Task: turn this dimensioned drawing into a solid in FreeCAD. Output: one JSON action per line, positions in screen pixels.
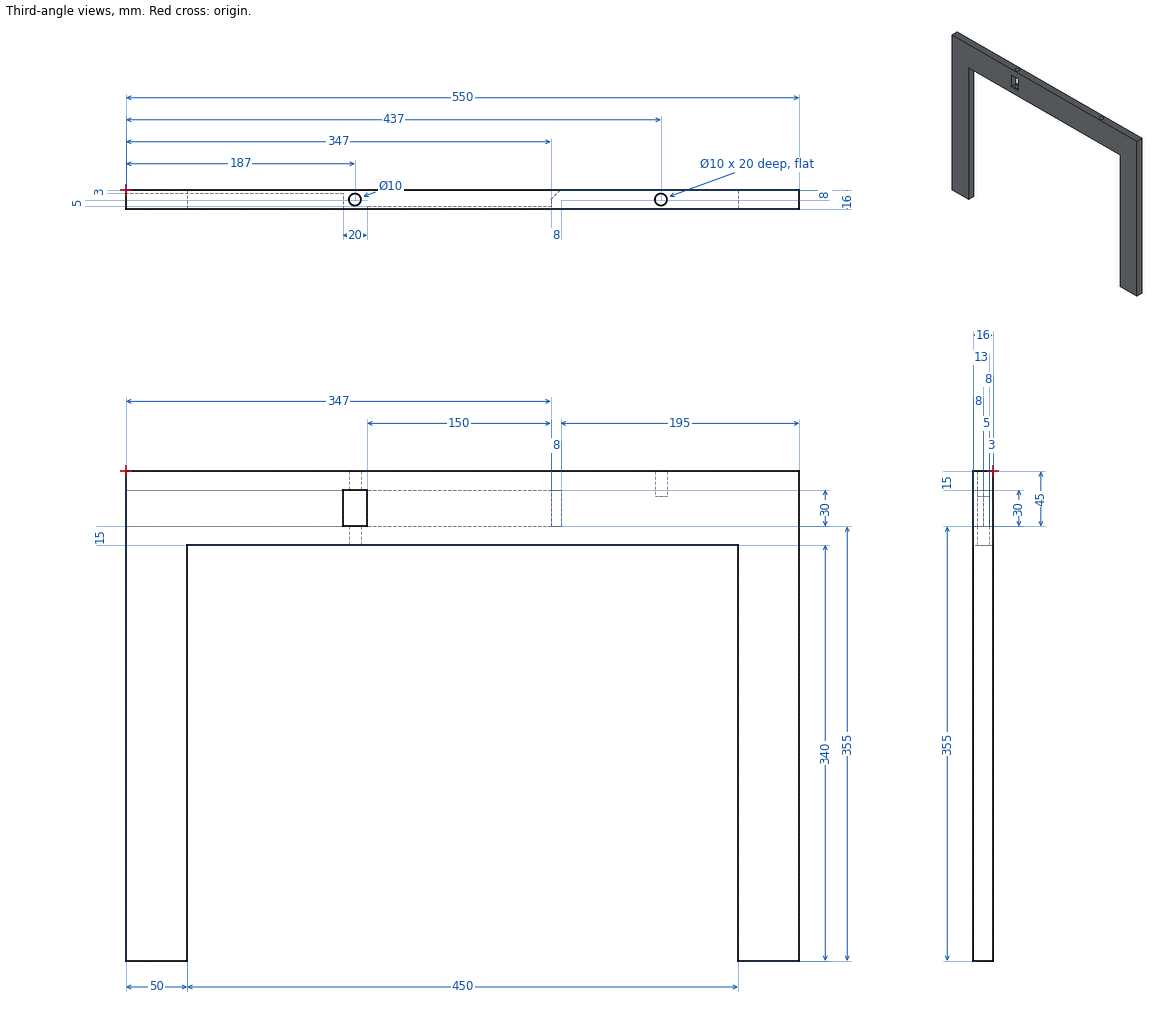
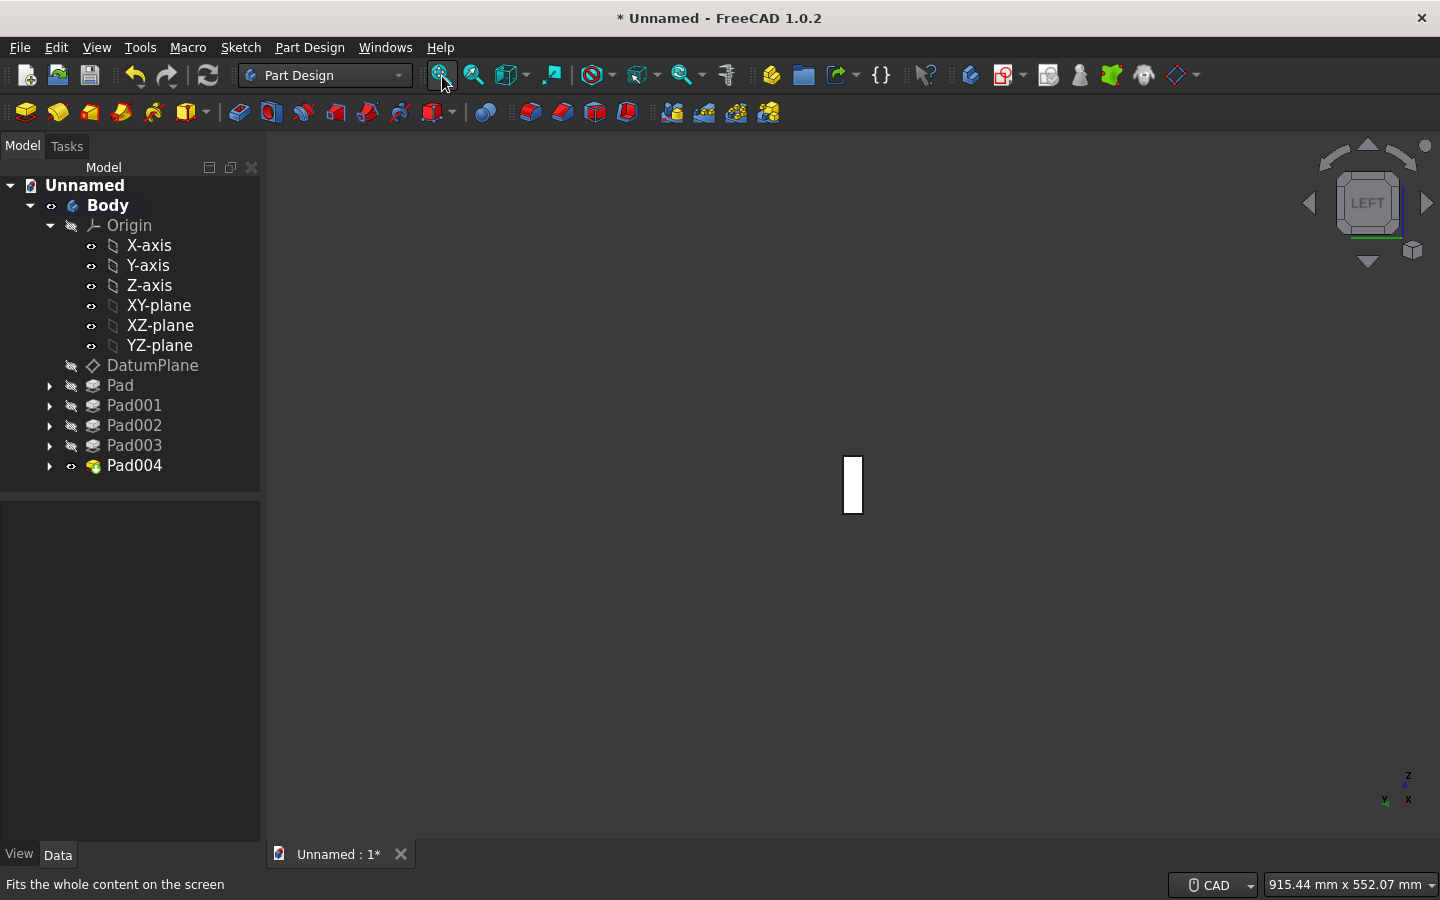
{"action": "key", "text": "4"}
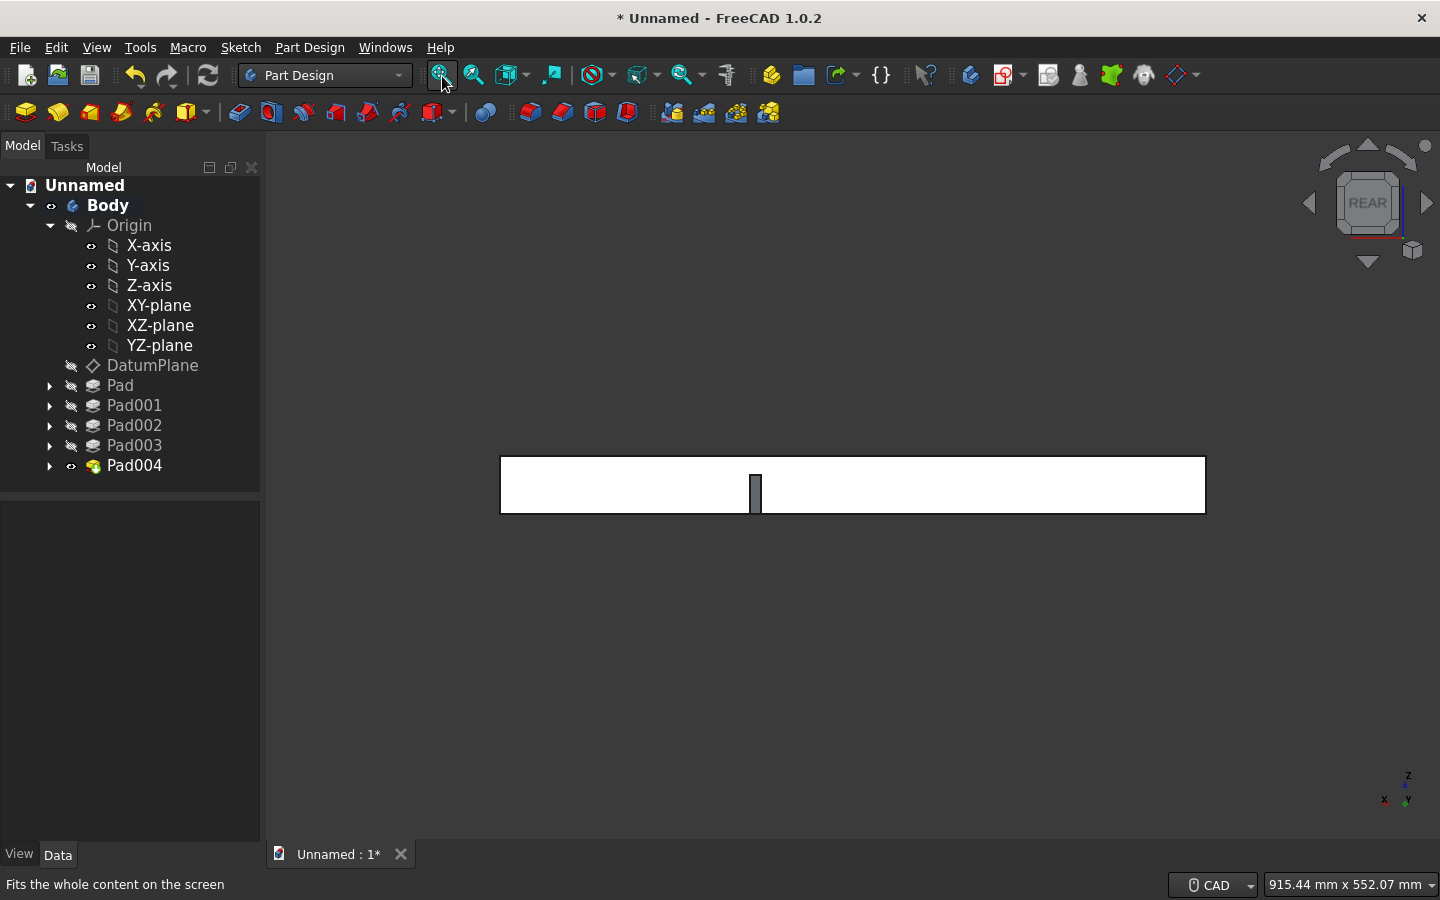
{"action": "left_click", "coordinate": [551, 484]}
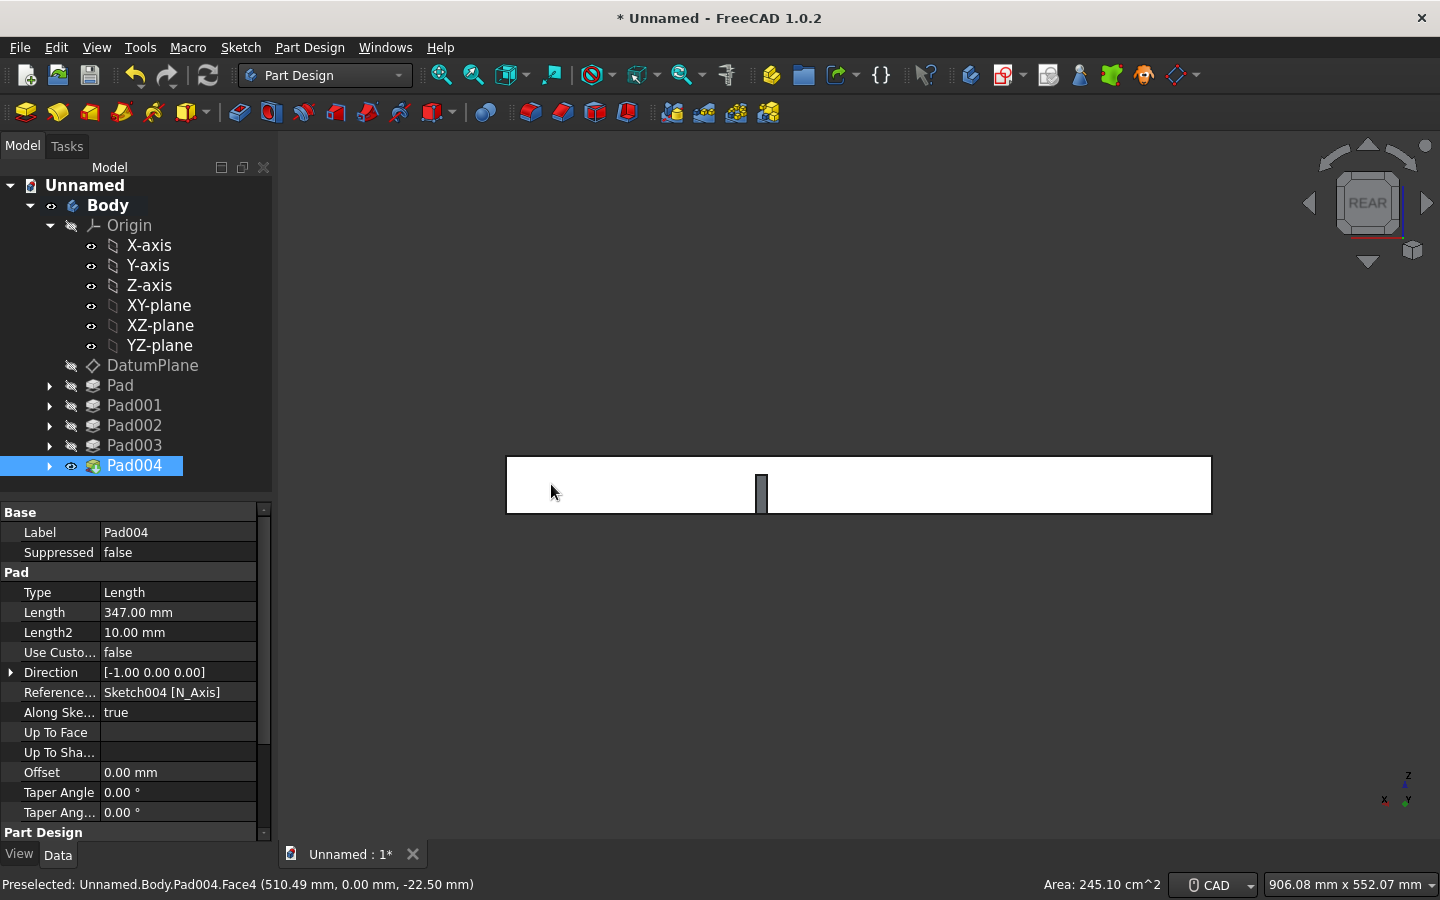
{"action": "left_click", "coordinate": [1004, 76]}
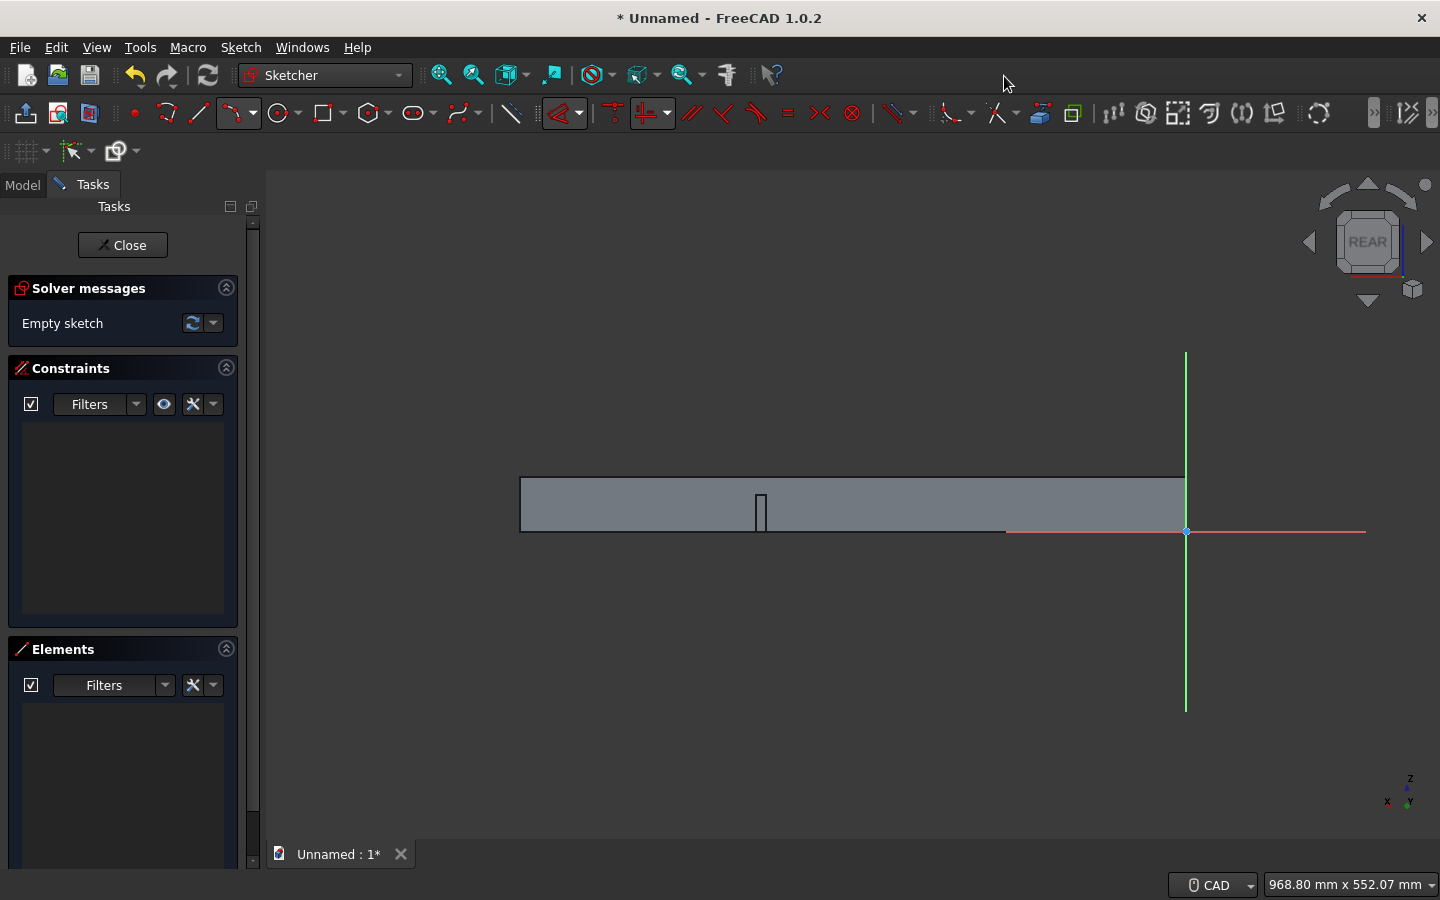
{"action": "scroll", "coordinate": [1275, 532], "scroll_direction": "up", "scroll_amount": 2}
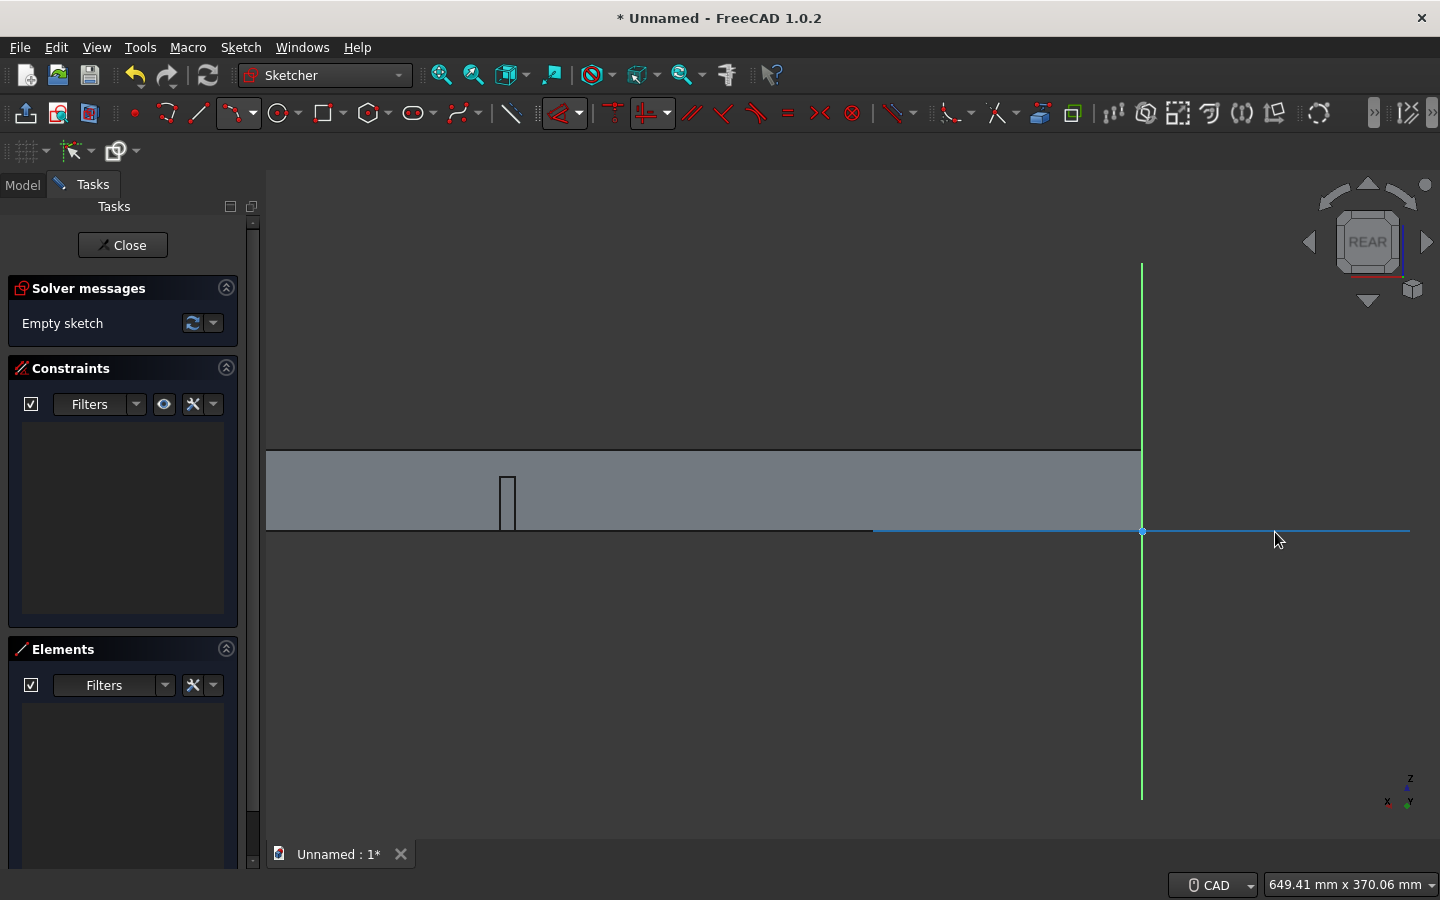
{"action": "left_click", "coordinate": [324, 114]}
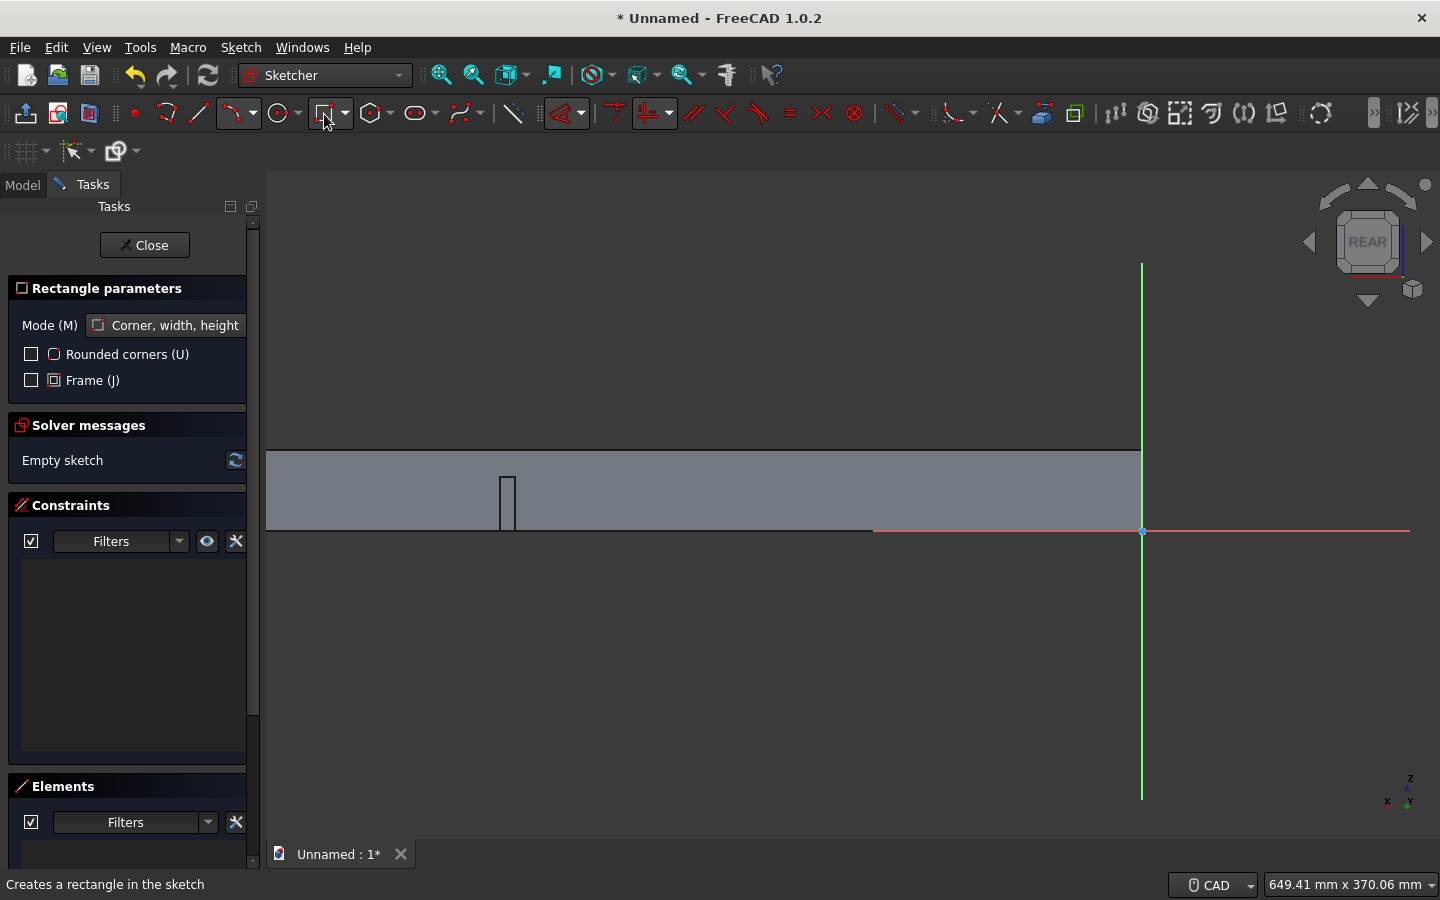
{"action": "left_click", "coordinate": [1142, 531]}
{"action": "left_click", "coordinate": [515, 477]}
{"action": "key", "text": "Escape"}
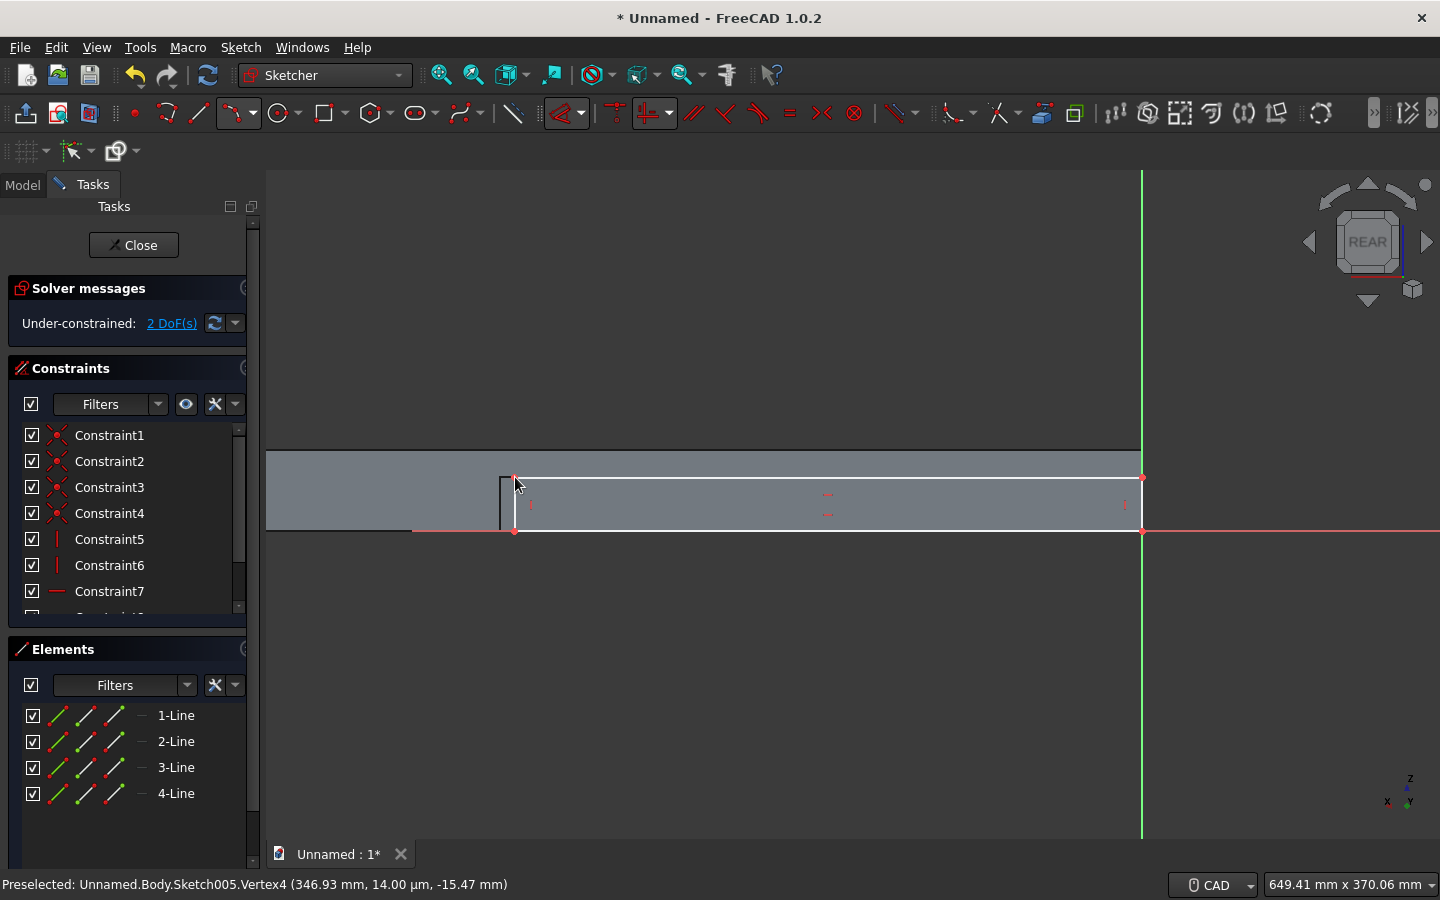
{"action": "left_click", "coordinate": [1142, 515]}